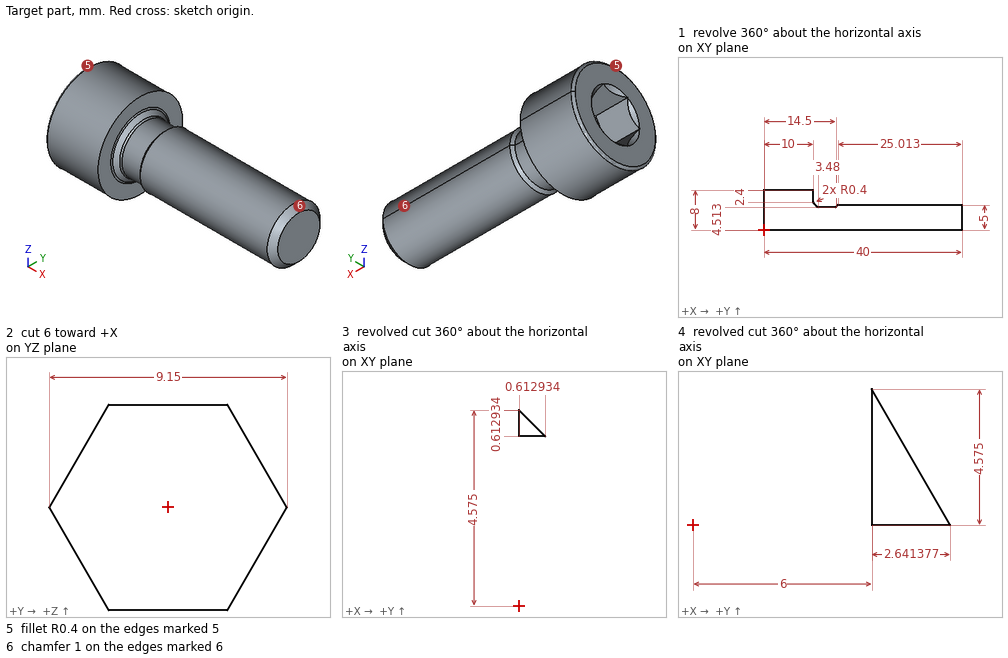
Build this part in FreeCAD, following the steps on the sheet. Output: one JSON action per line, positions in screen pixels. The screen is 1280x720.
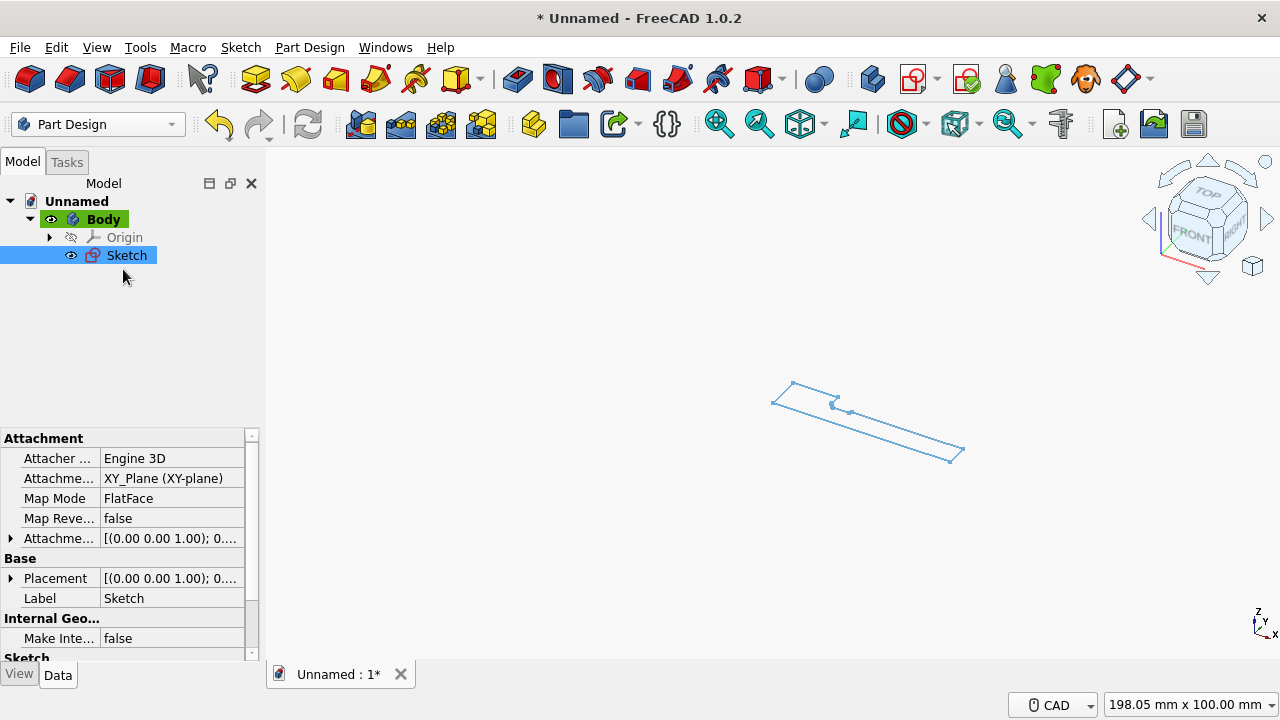
{"action": "left_click", "coordinate": [296, 80]}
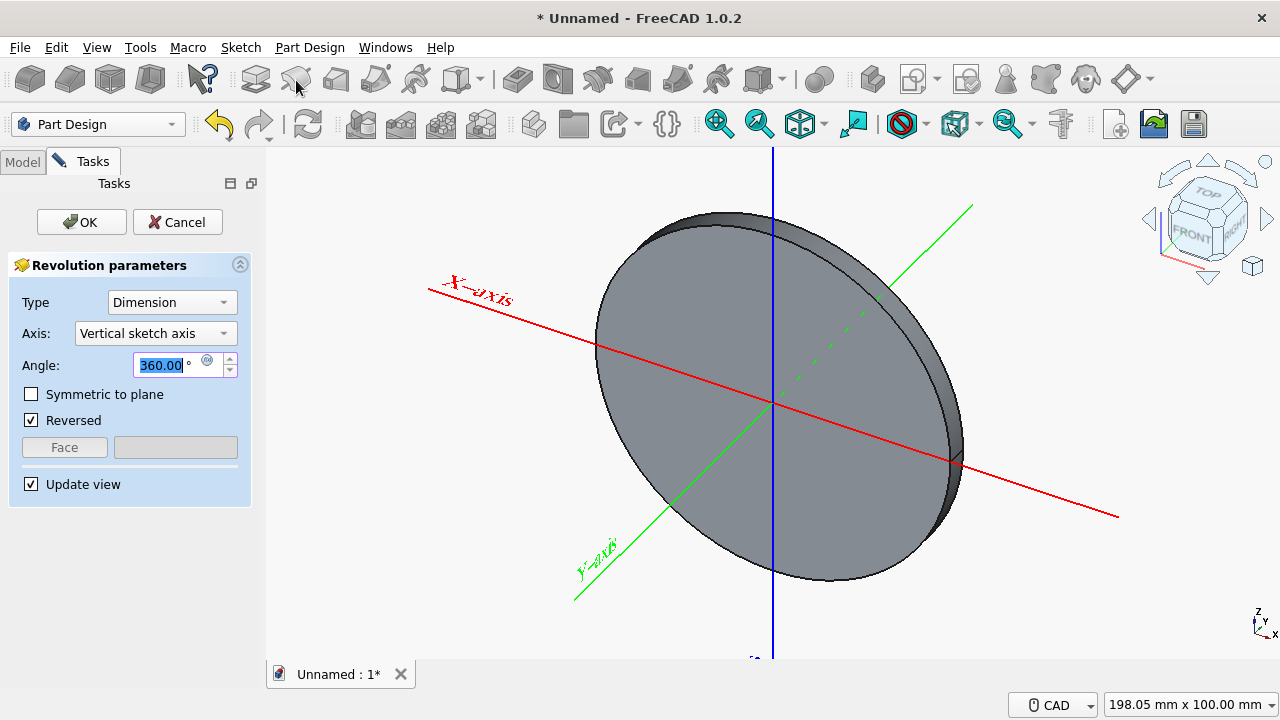
{"action": "left_click", "coordinate": [156, 334]}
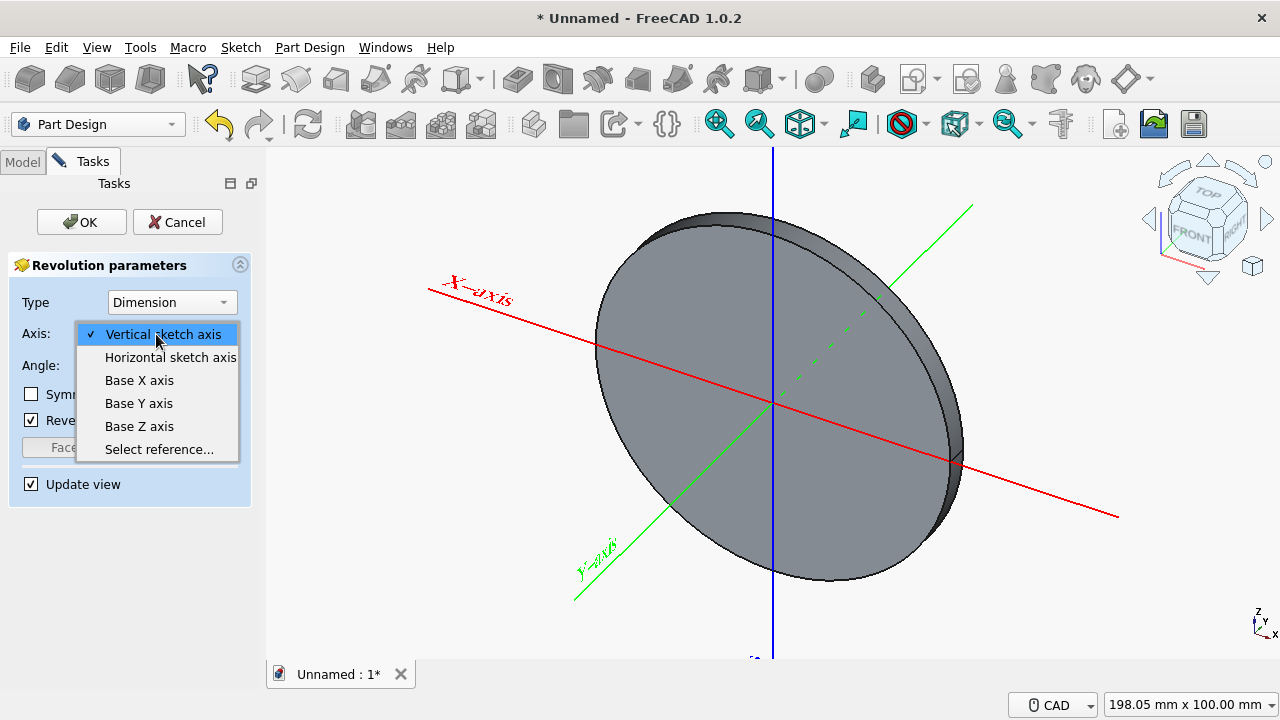
{"action": "left_click", "coordinate": [156, 358]}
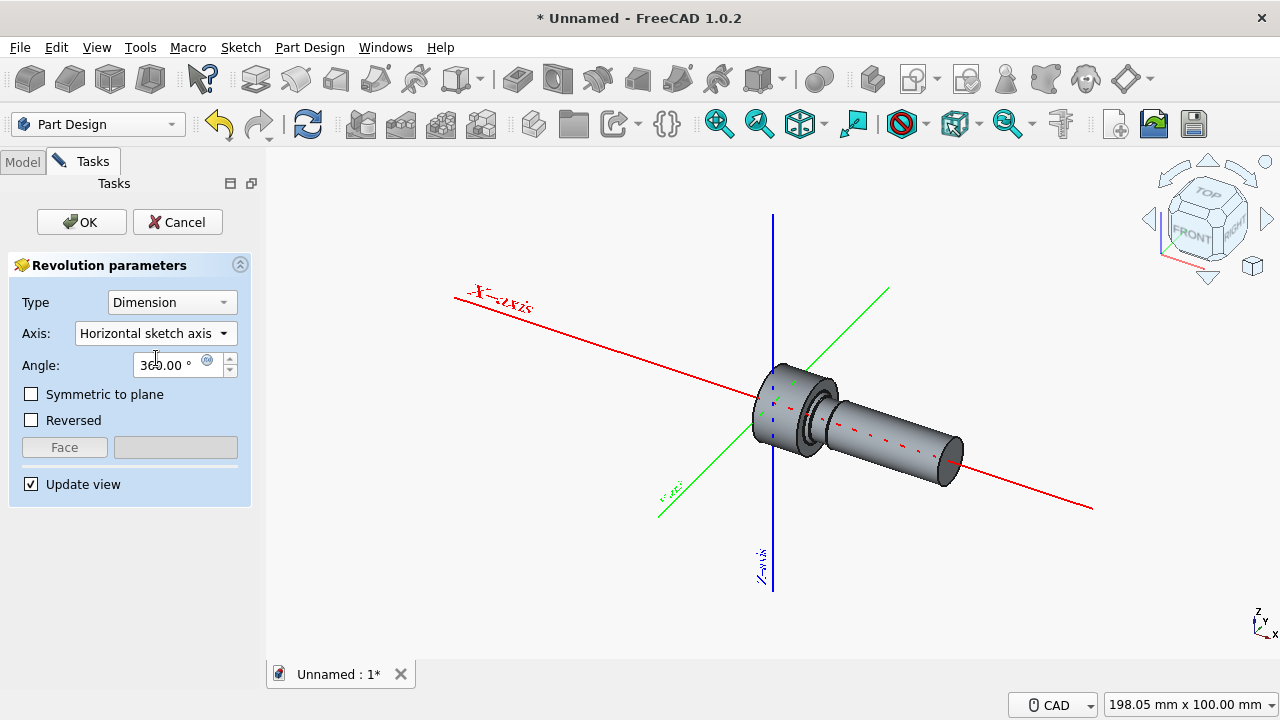
{"action": "left_click", "coordinate": [82, 222]}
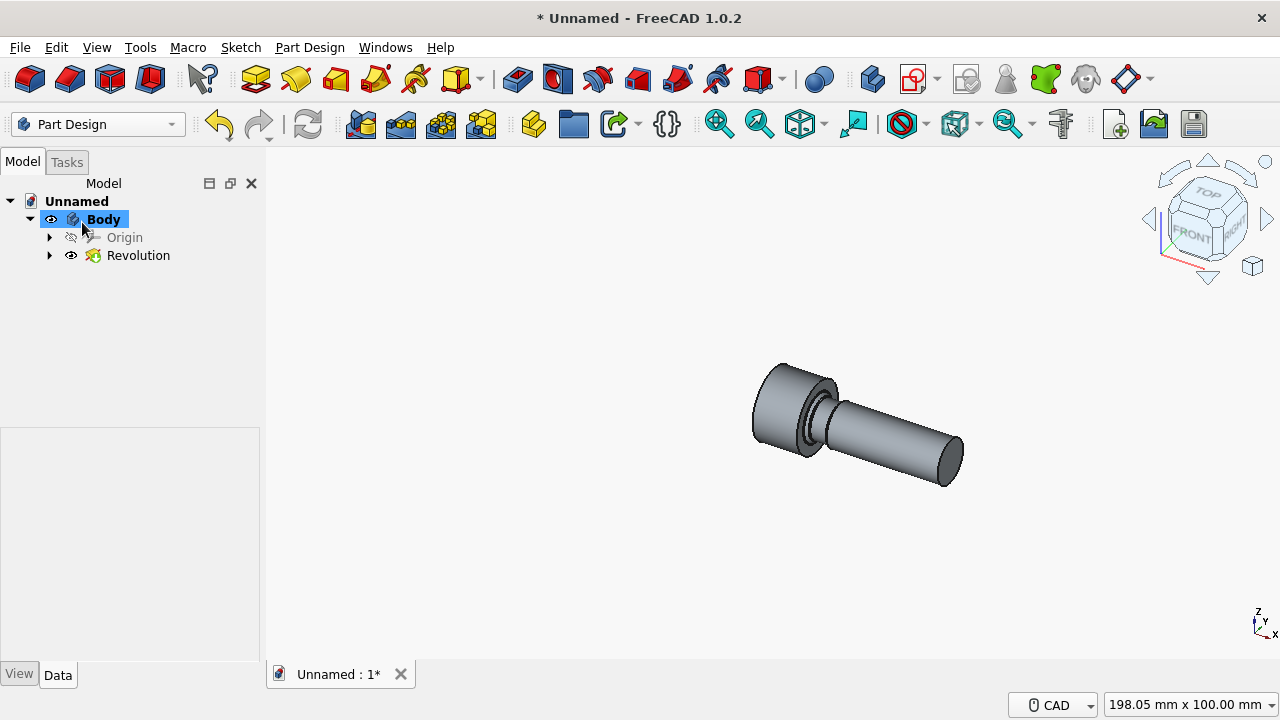
{"action": "left_click", "coordinate": [720, 124]}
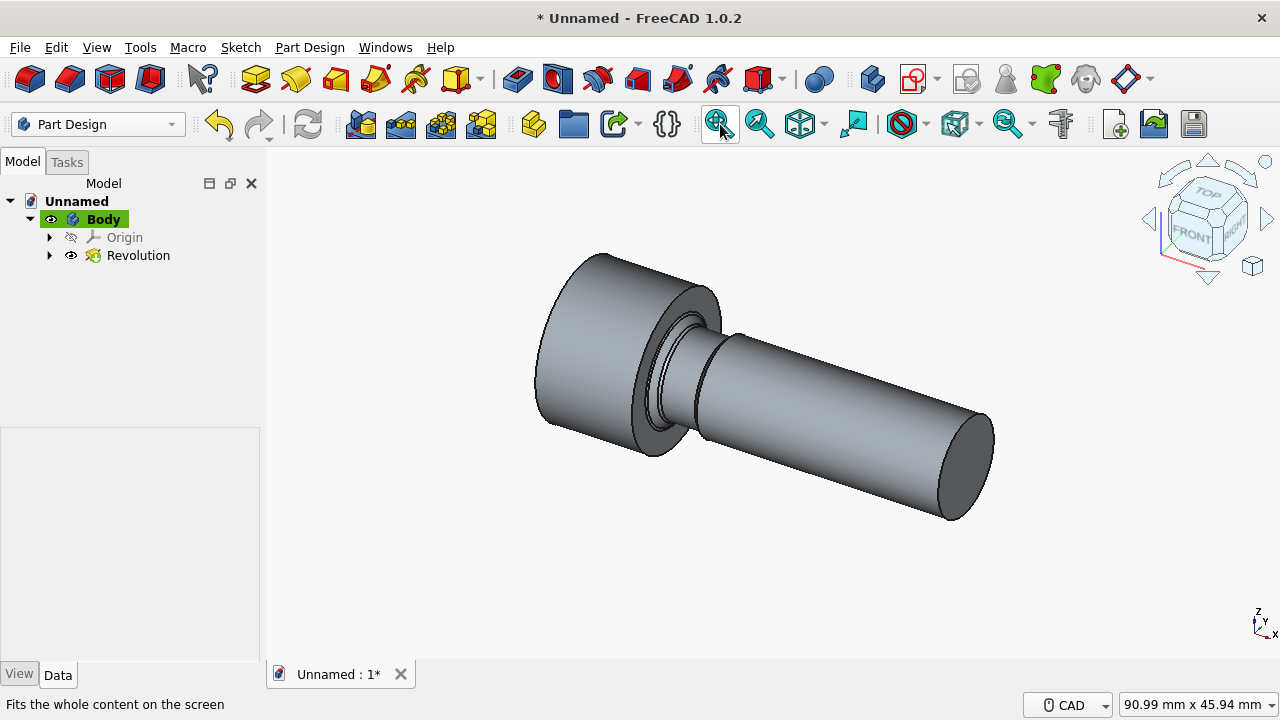
{"action": "left_click", "coordinate": [914, 80]}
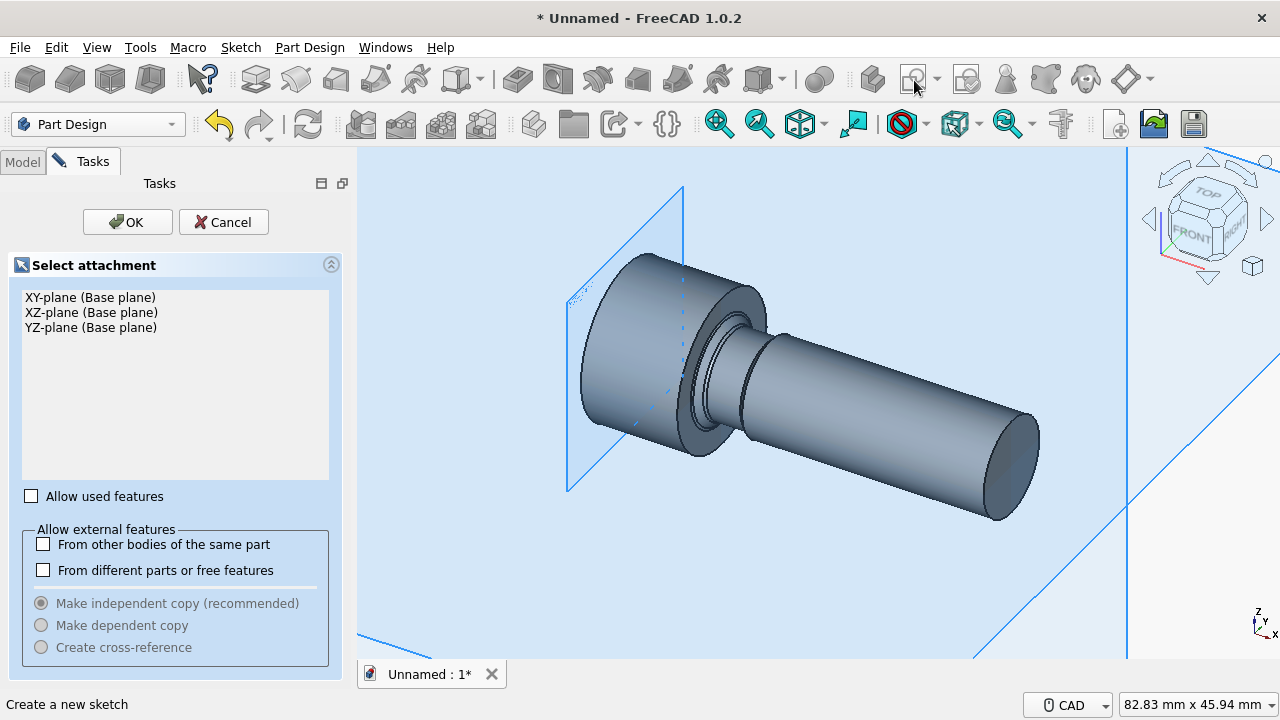
{"action": "left_click", "coordinate": [82, 328]}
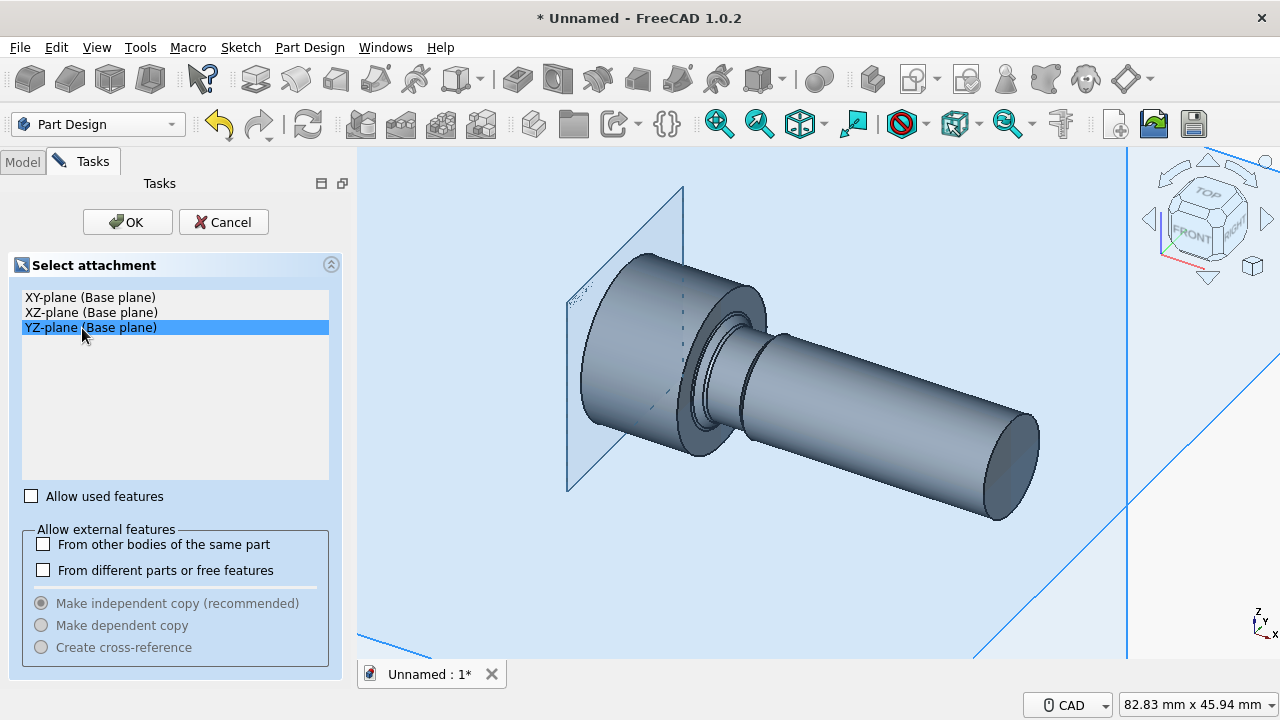
{"action": "left_click", "coordinate": [128, 222]}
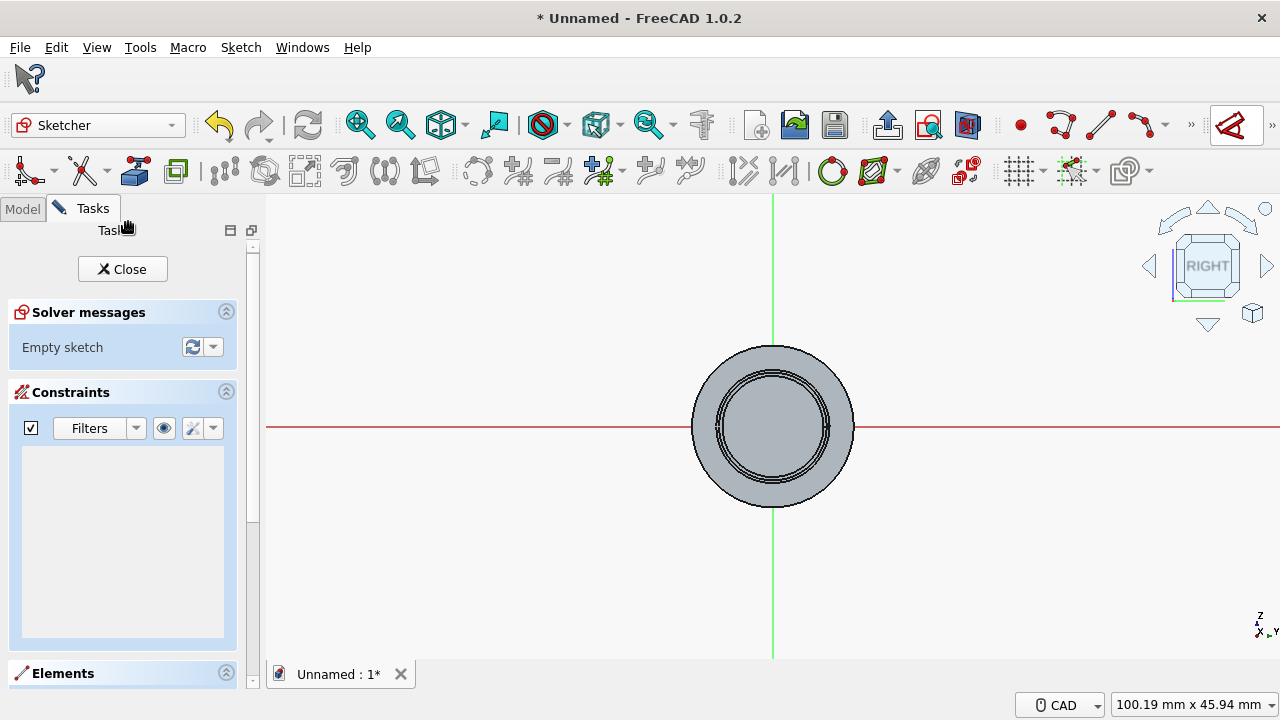
{"action": "left_click", "coordinate": [968, 126]}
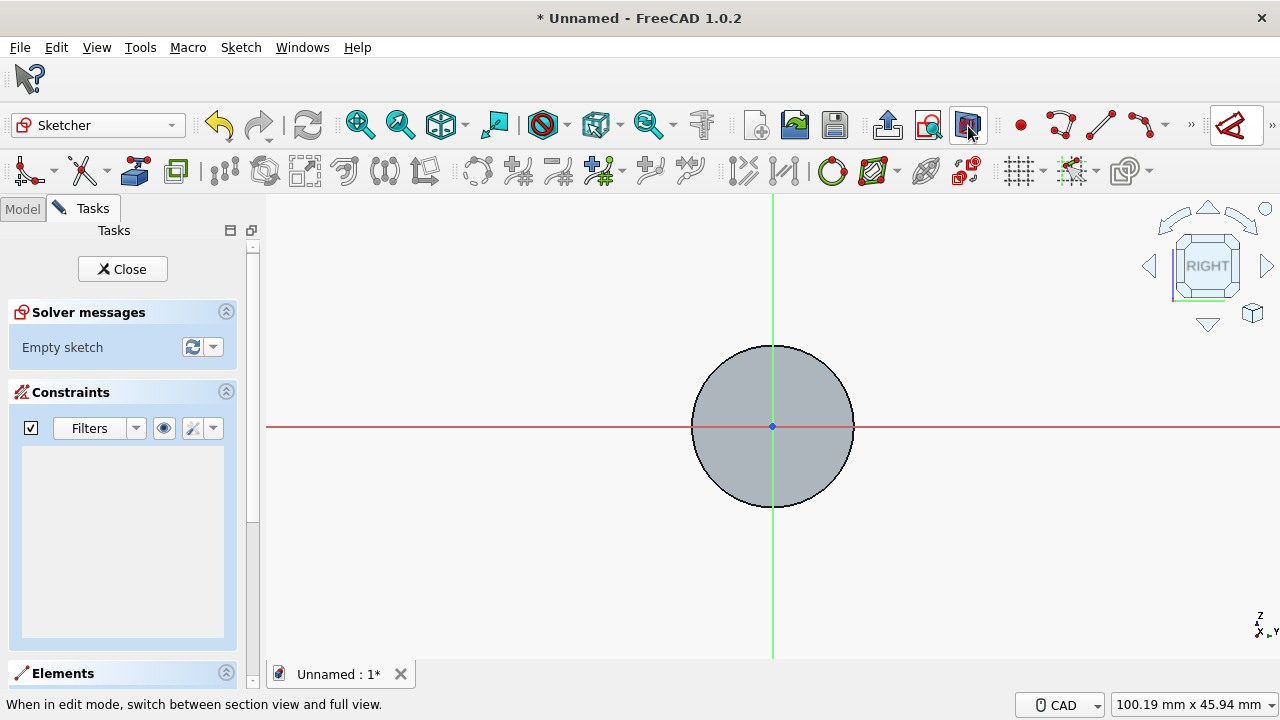
{"action": "scroll", "coordinate": [802, 427], "scroll_direction": "up", "scroll_amount": 6}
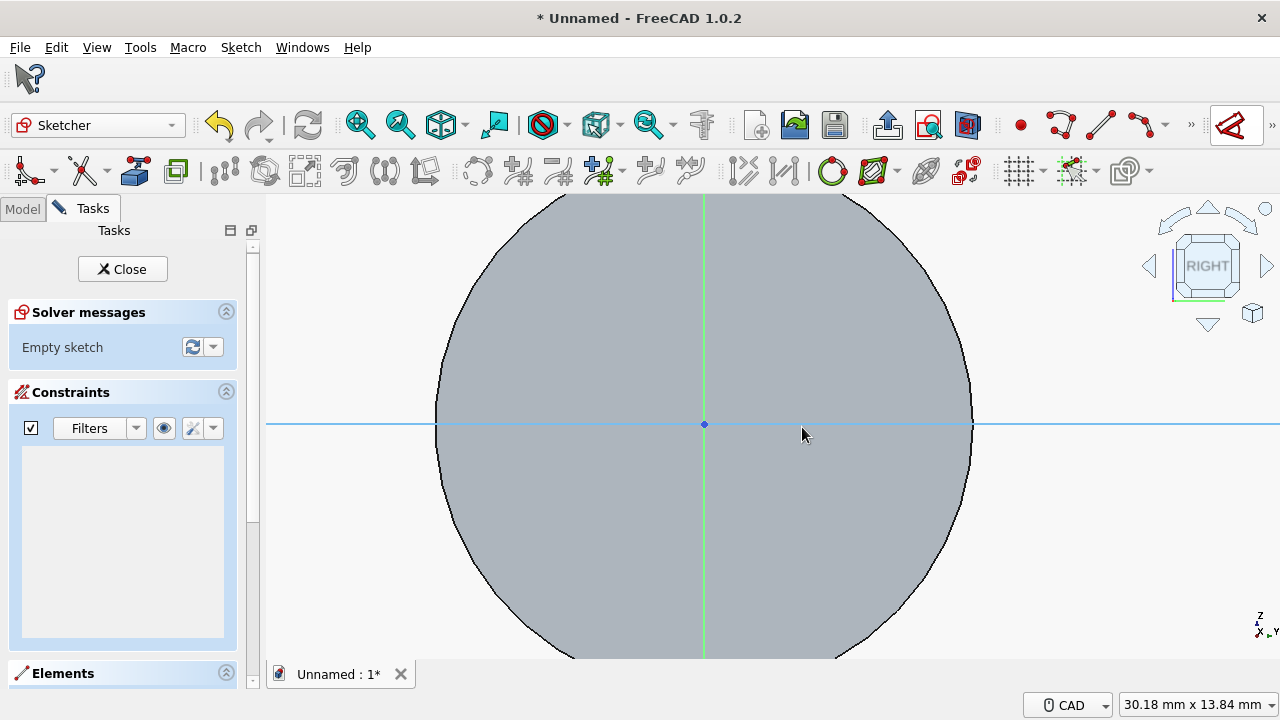
{"action": "key", "text": "g p 6"}